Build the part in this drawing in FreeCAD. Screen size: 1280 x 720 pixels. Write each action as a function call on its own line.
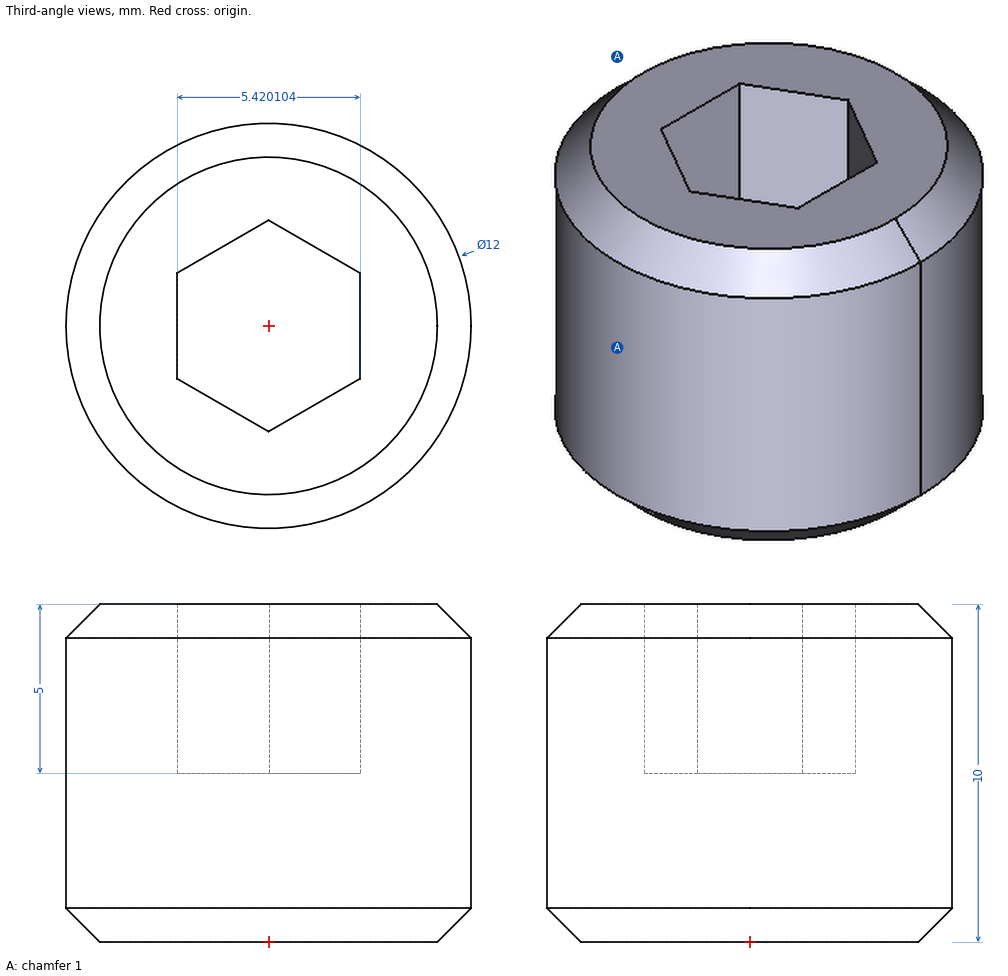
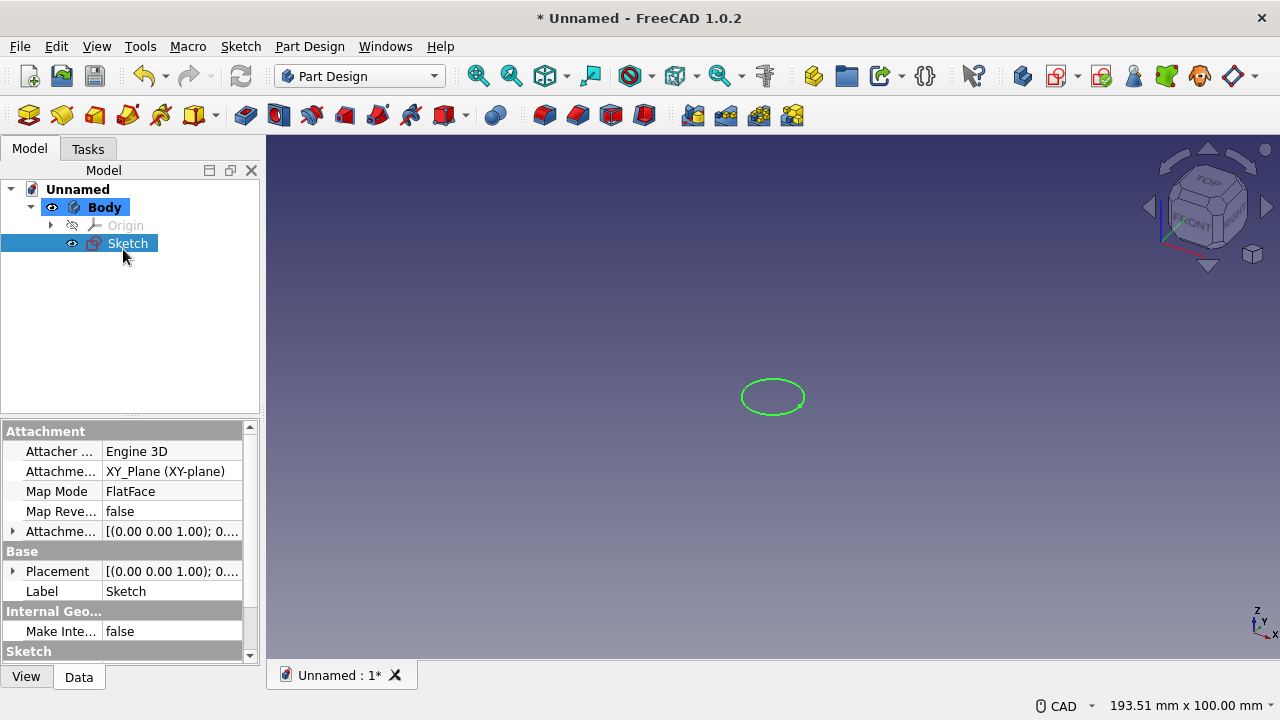
click(29, 116)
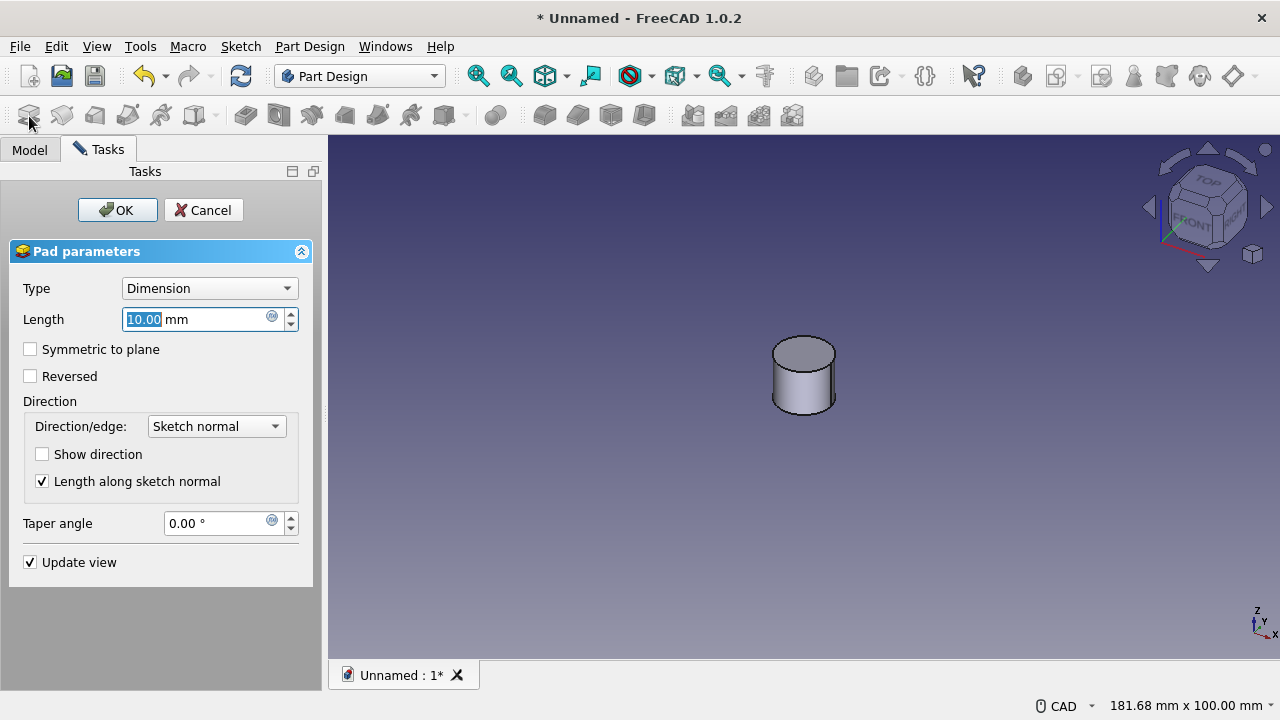
text(10)
key(Tab)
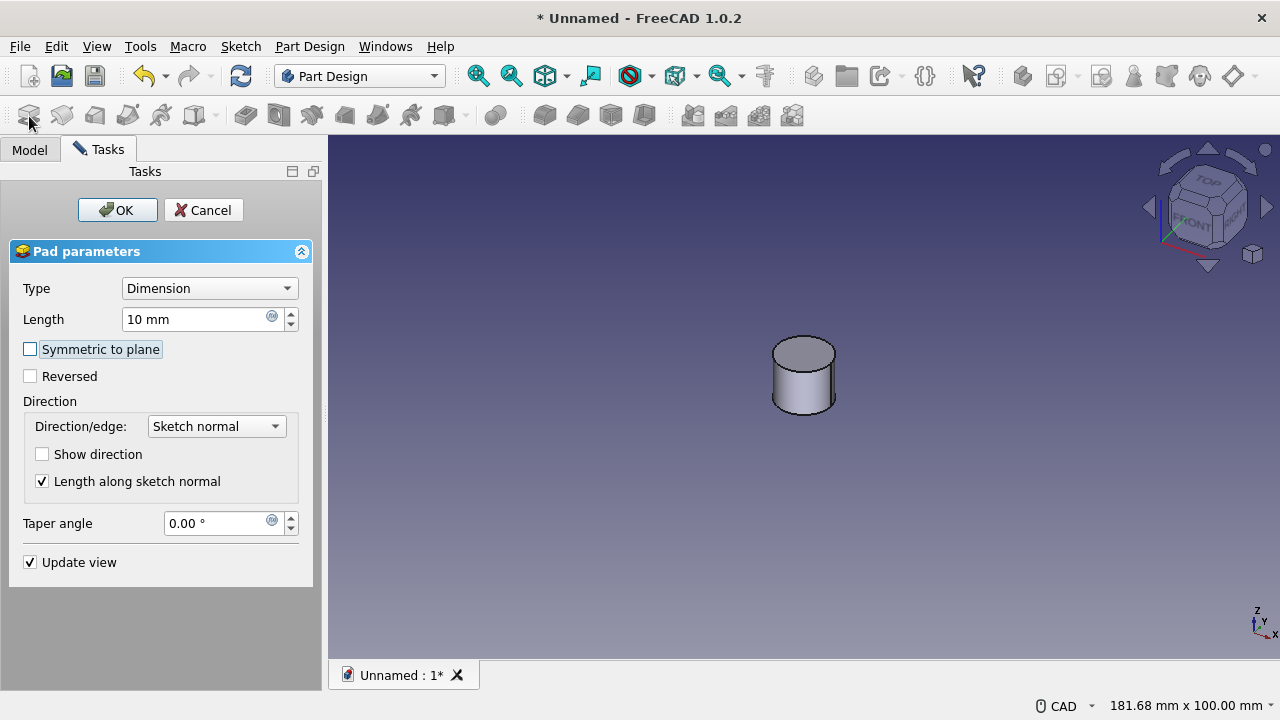
click(118, 210)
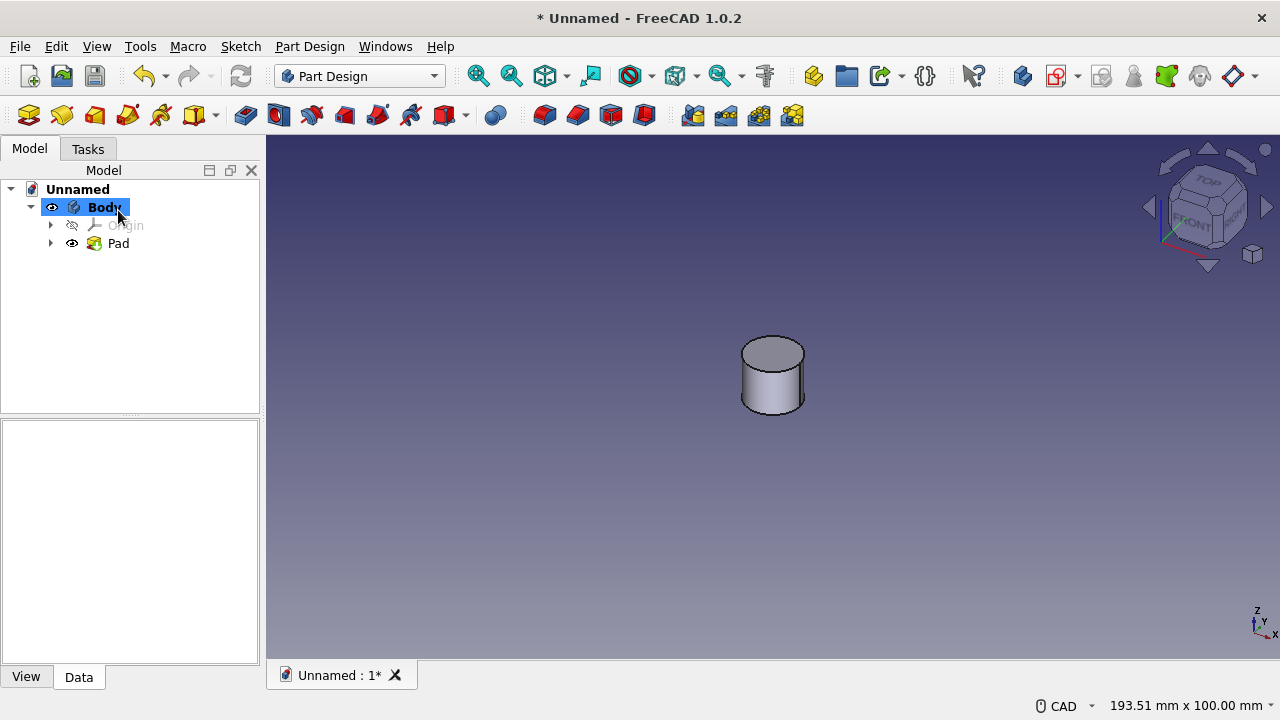
click(479, 76)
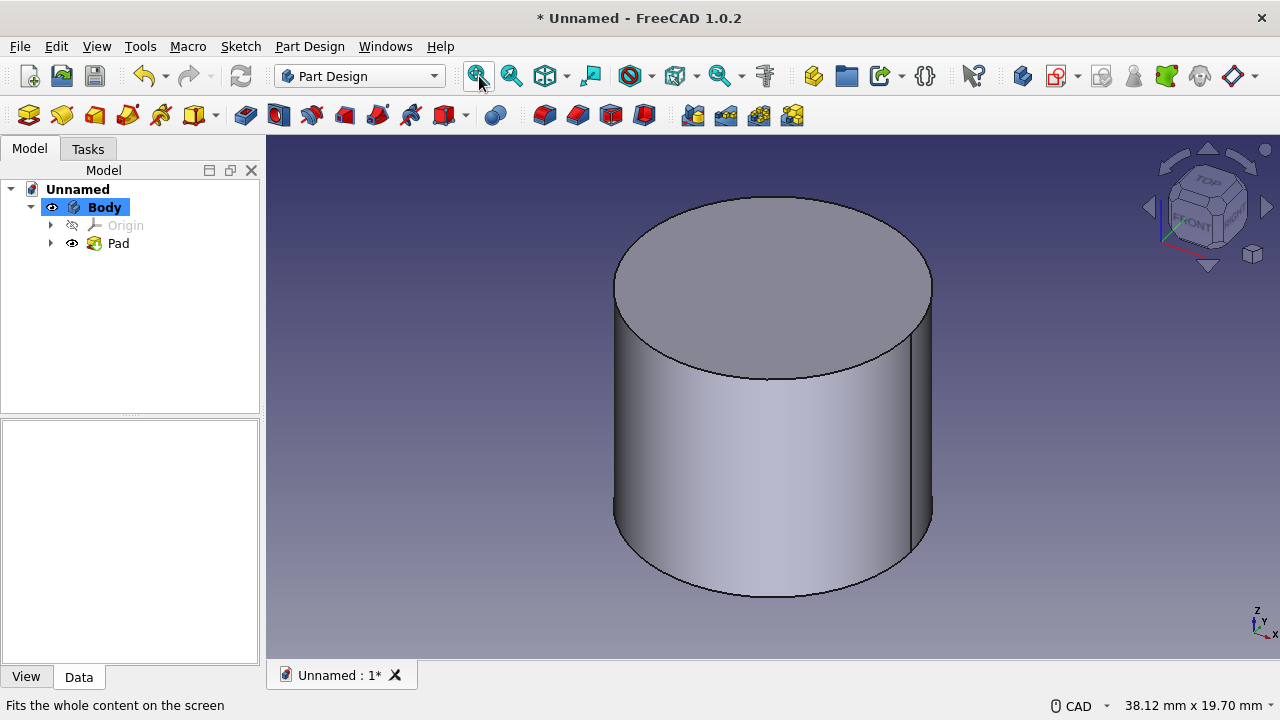
click(773, 287)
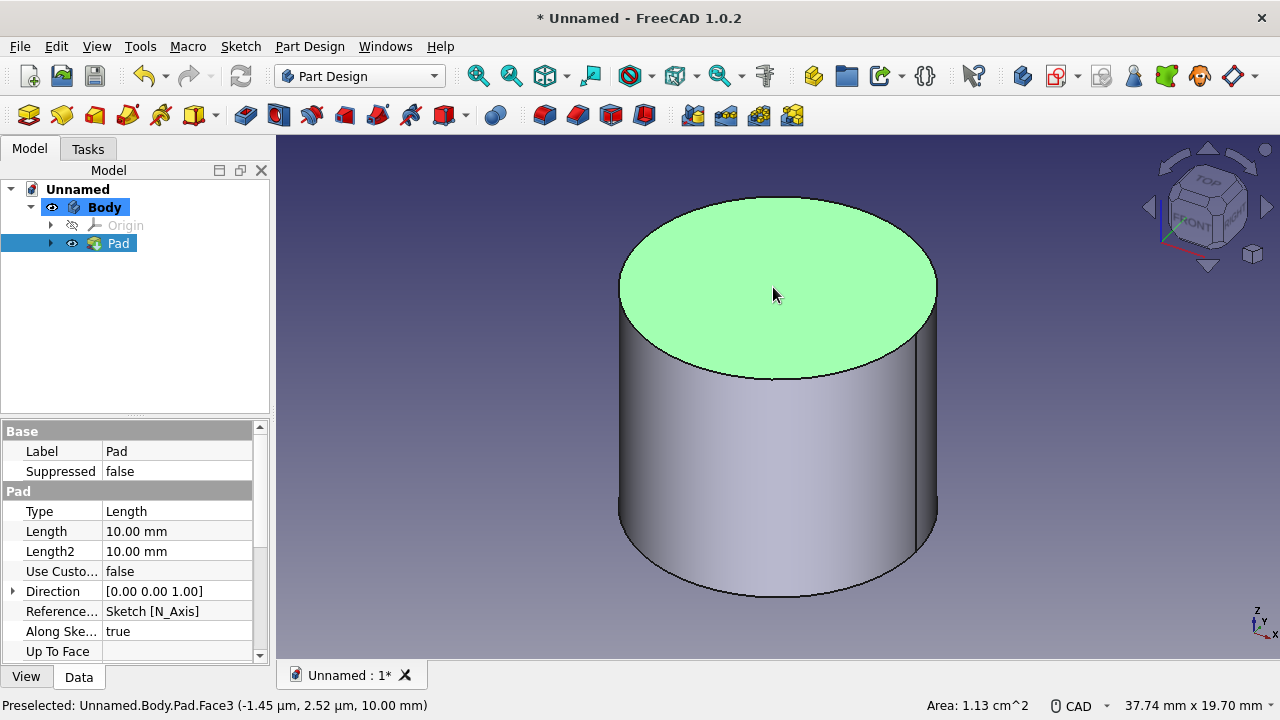
click(1056, 76)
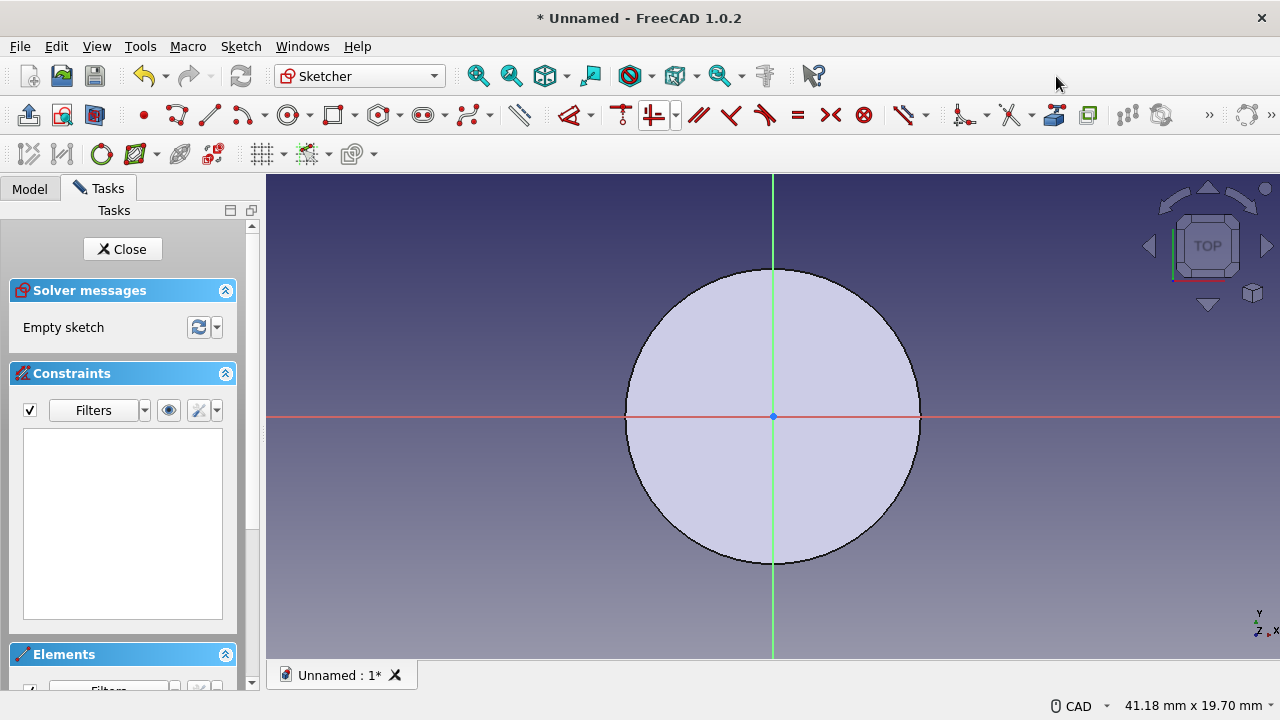
scroll(856, 416, up, 3)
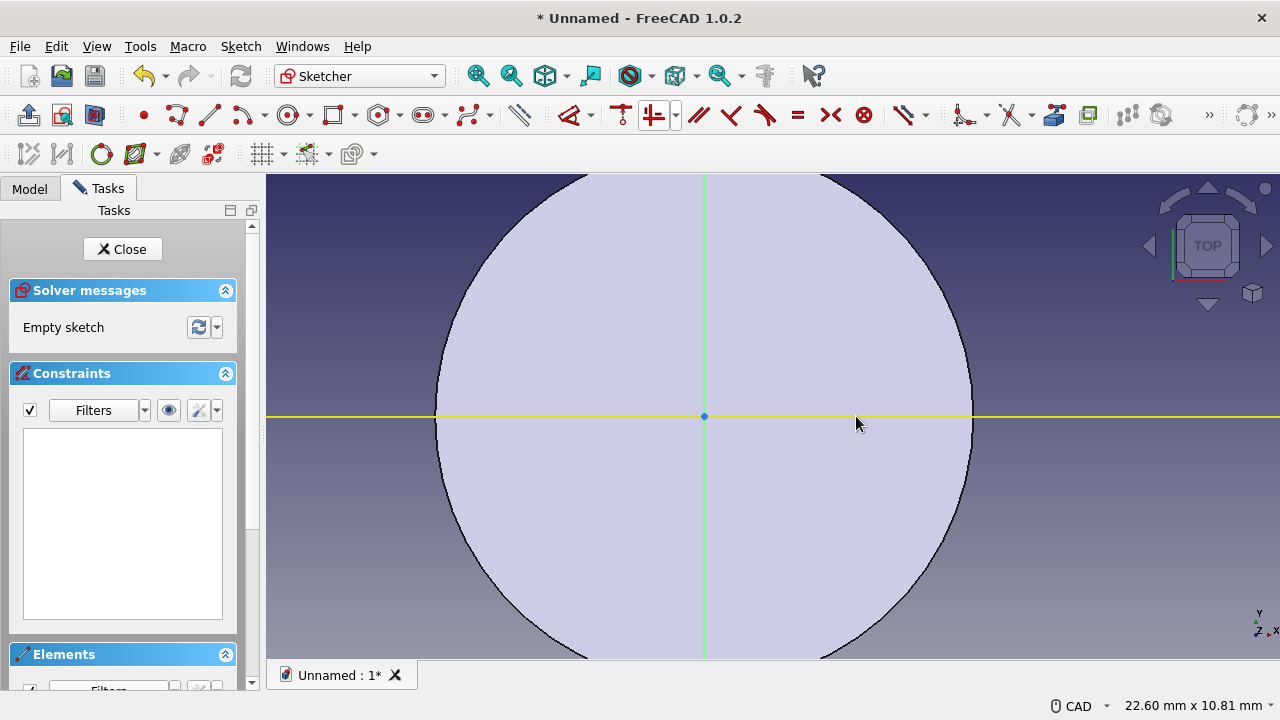
click(378, 116)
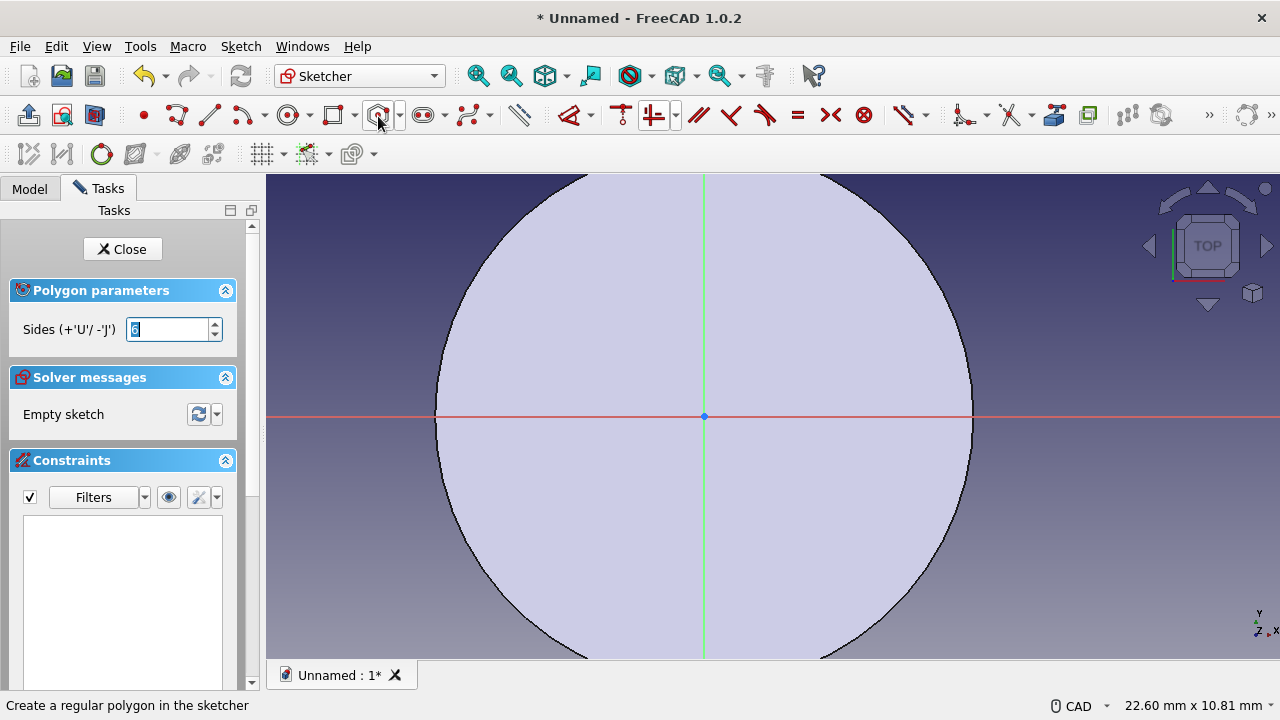
click(704, 416)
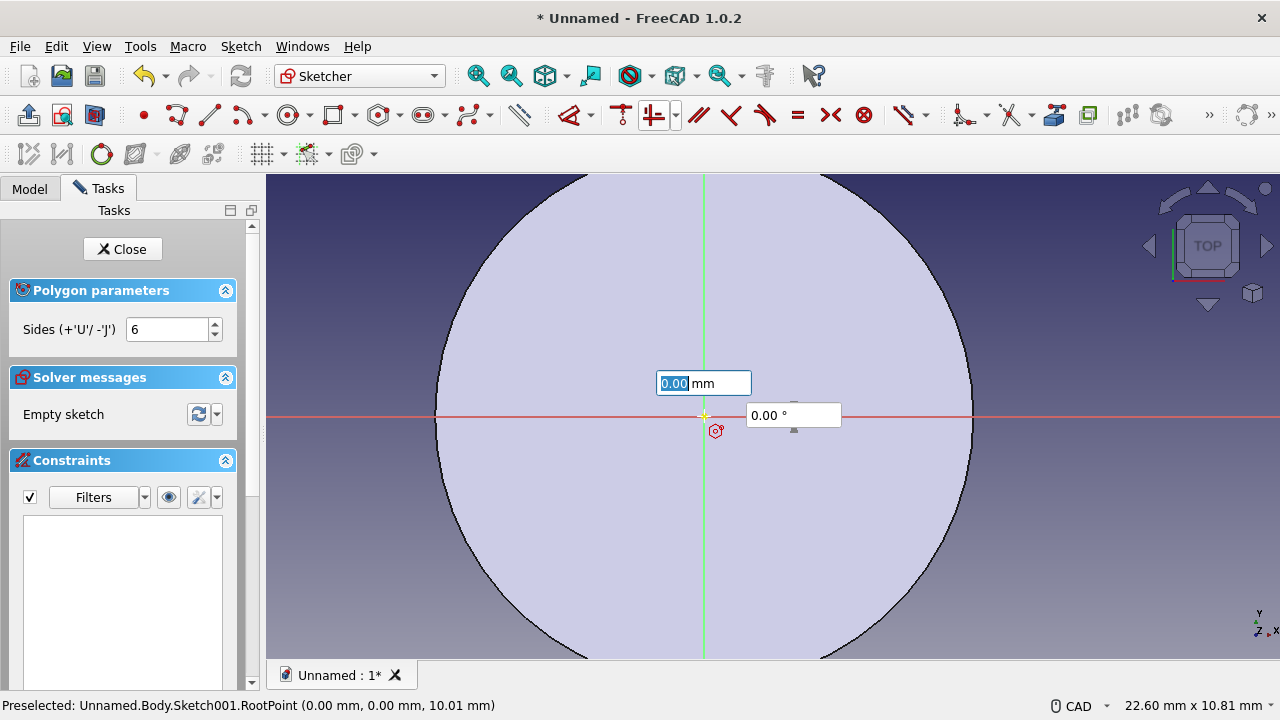
click(704, 276)
right_click(704, 276)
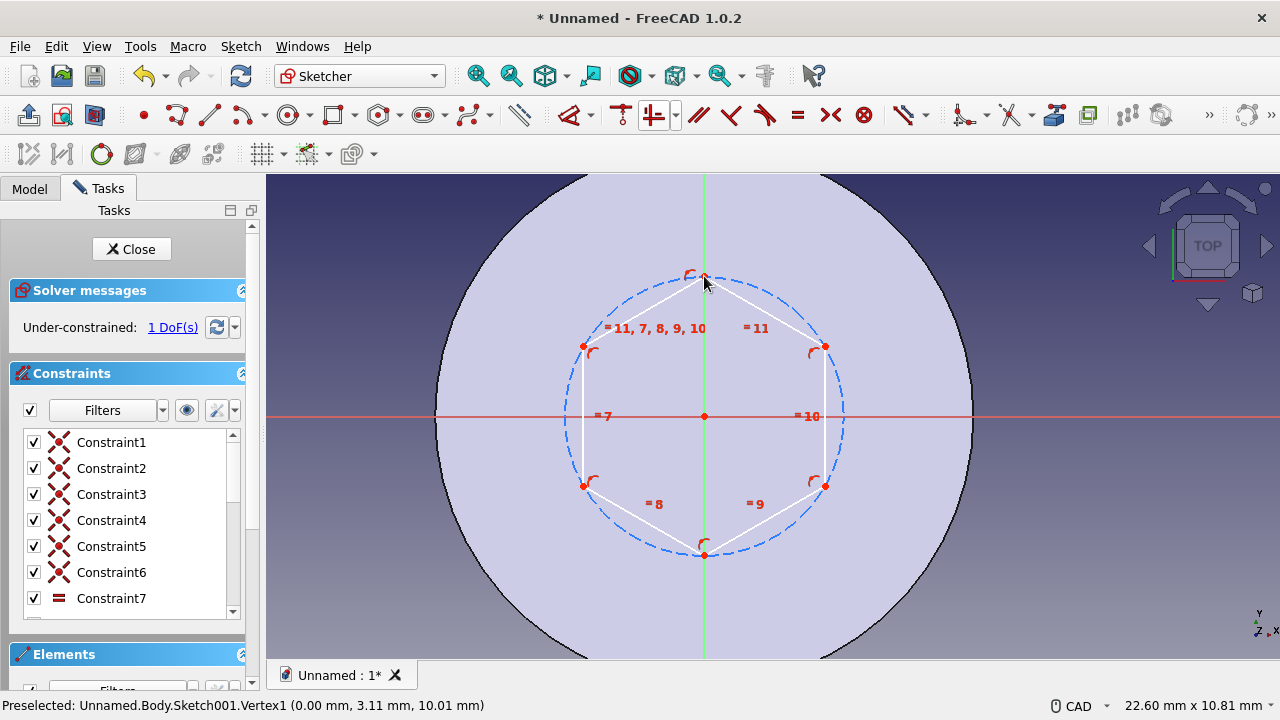
click(583, 347)